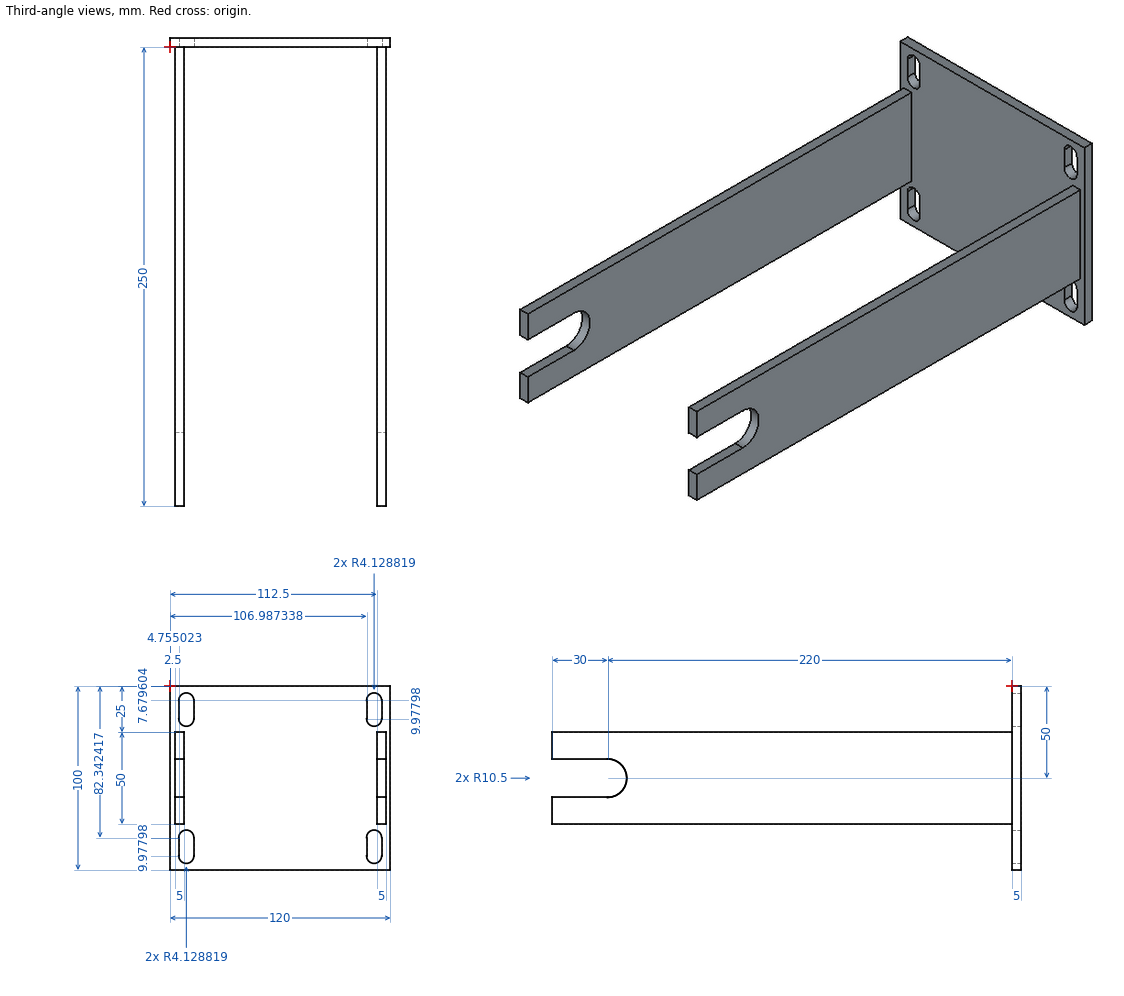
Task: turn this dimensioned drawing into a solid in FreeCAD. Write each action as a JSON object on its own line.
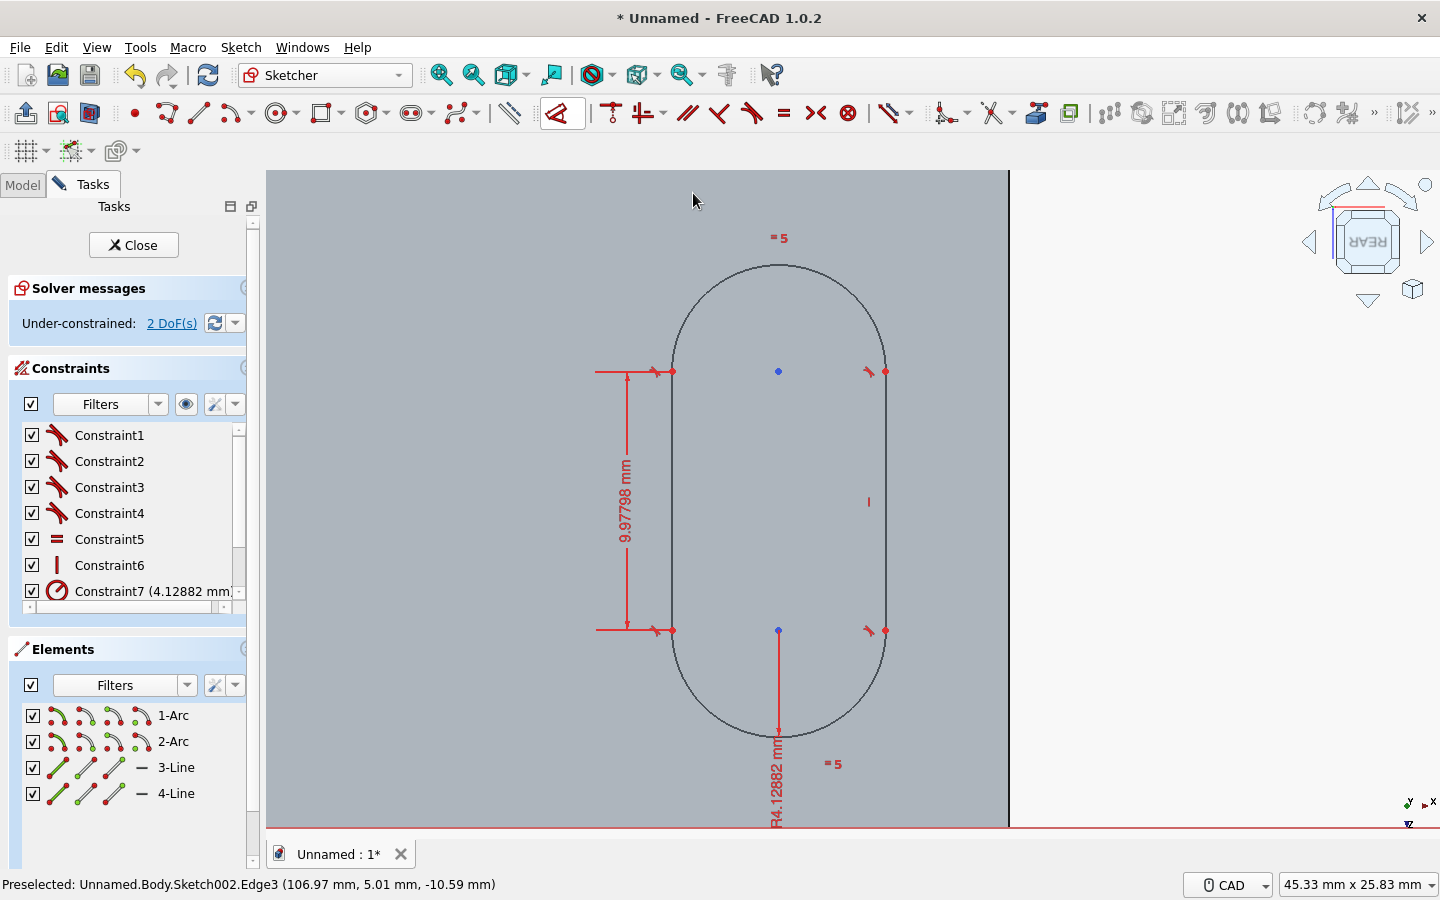
{"action": "left_click", "coordinate": [672, 630]}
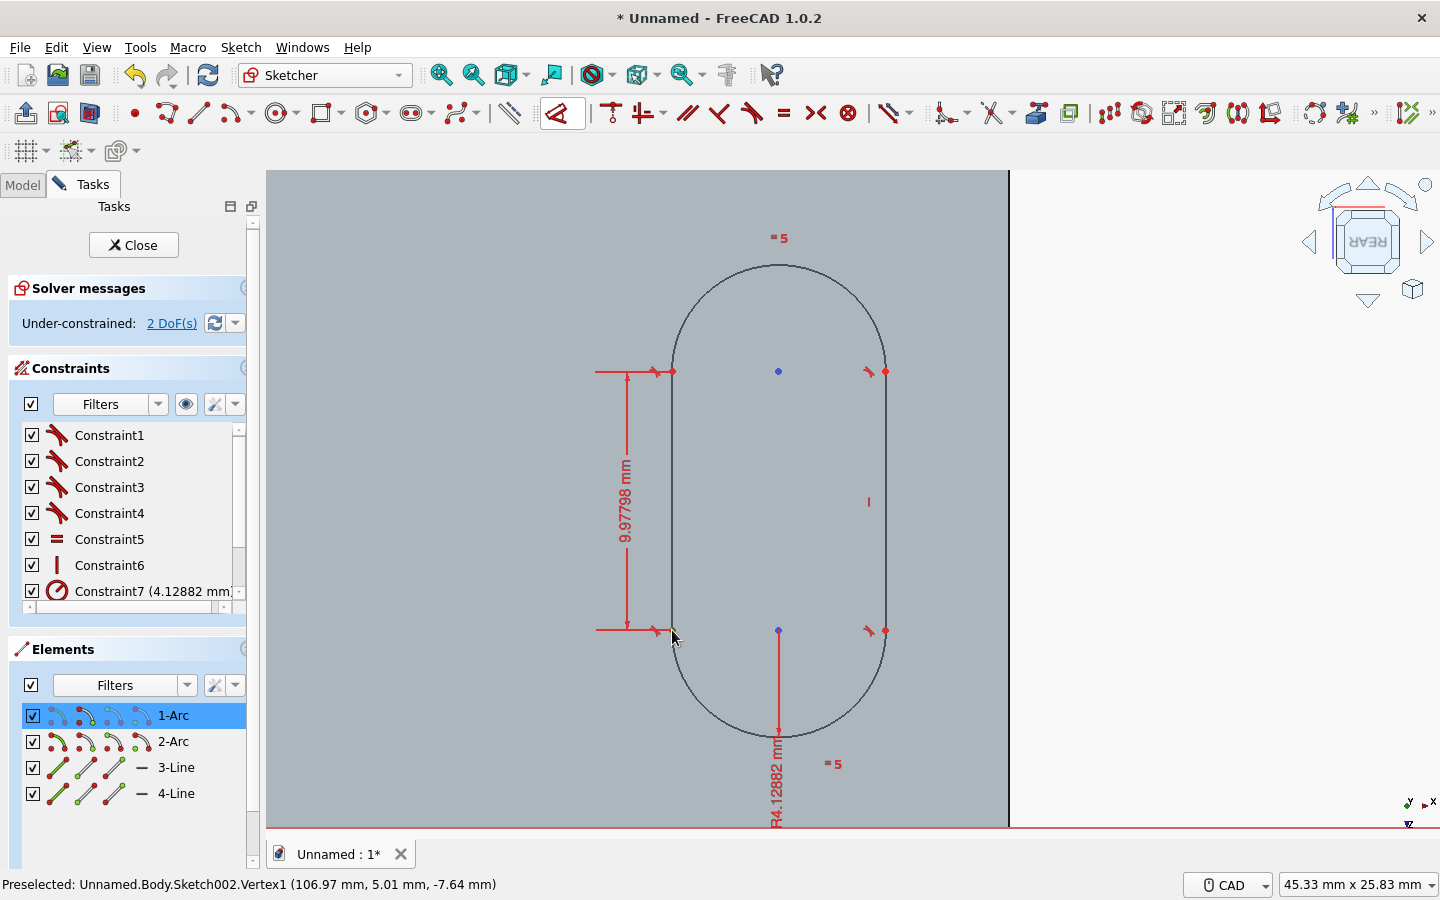
{"action": "left_click", "coordinate": [580, 114]}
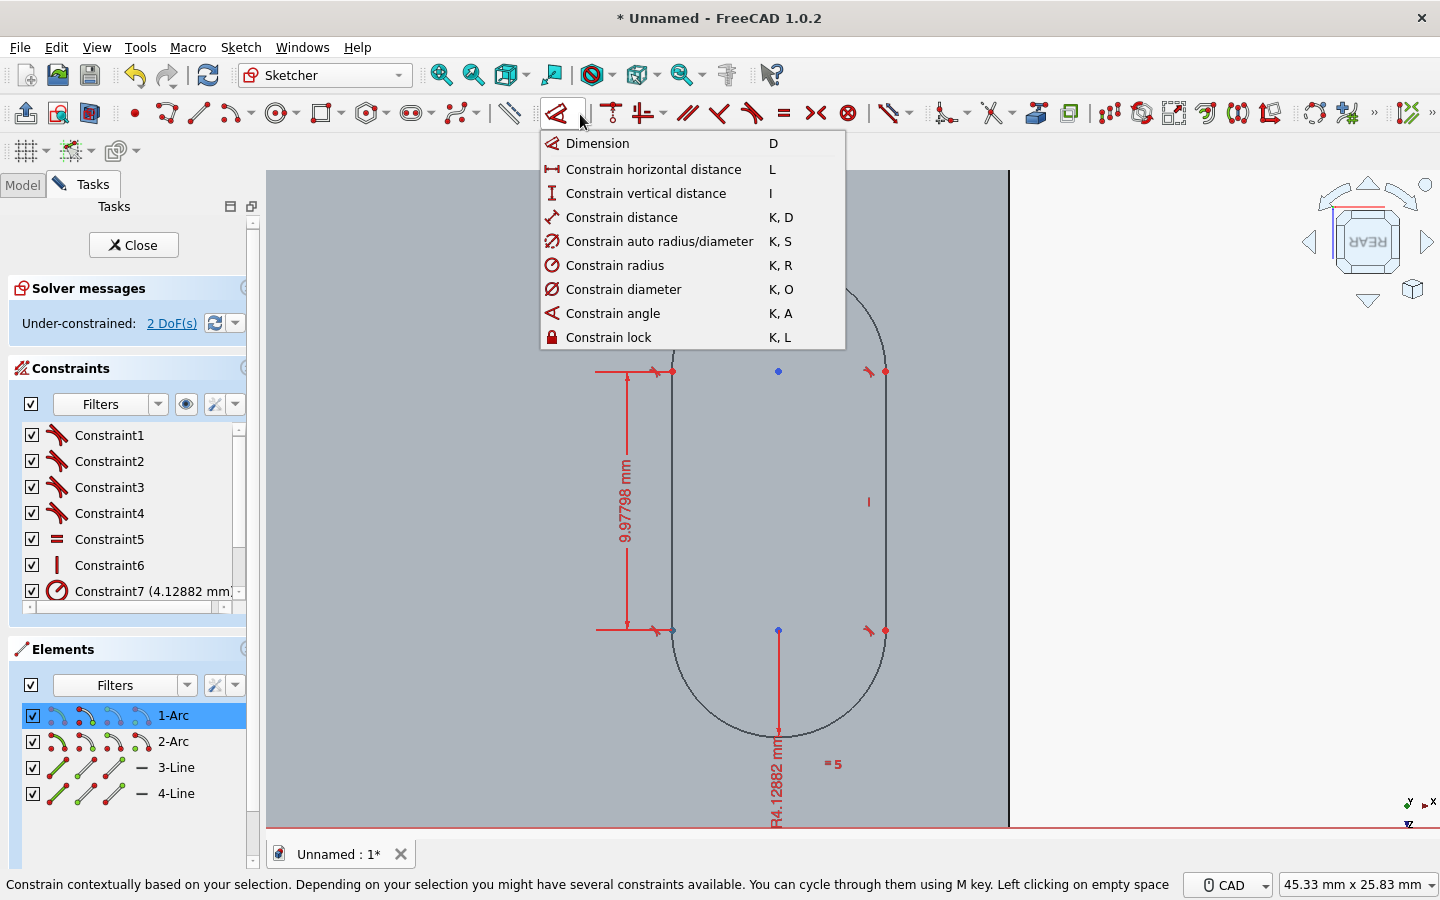
{"action": "left_click", "coordinate": [693, 193]}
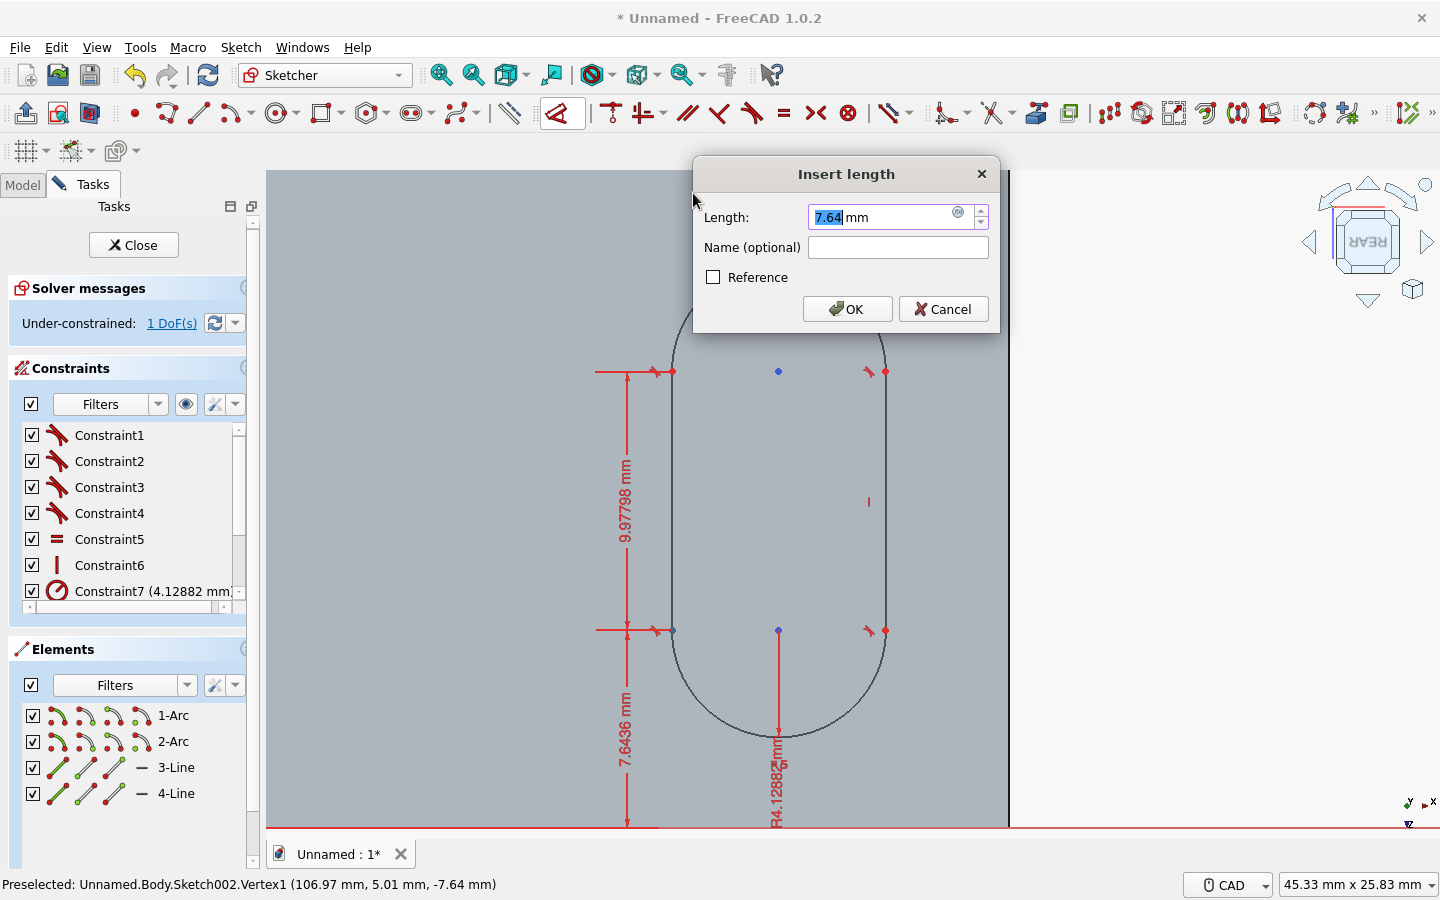
{"action": "type", "text": "7.679604"}
{"action": "key", "text": "Return"}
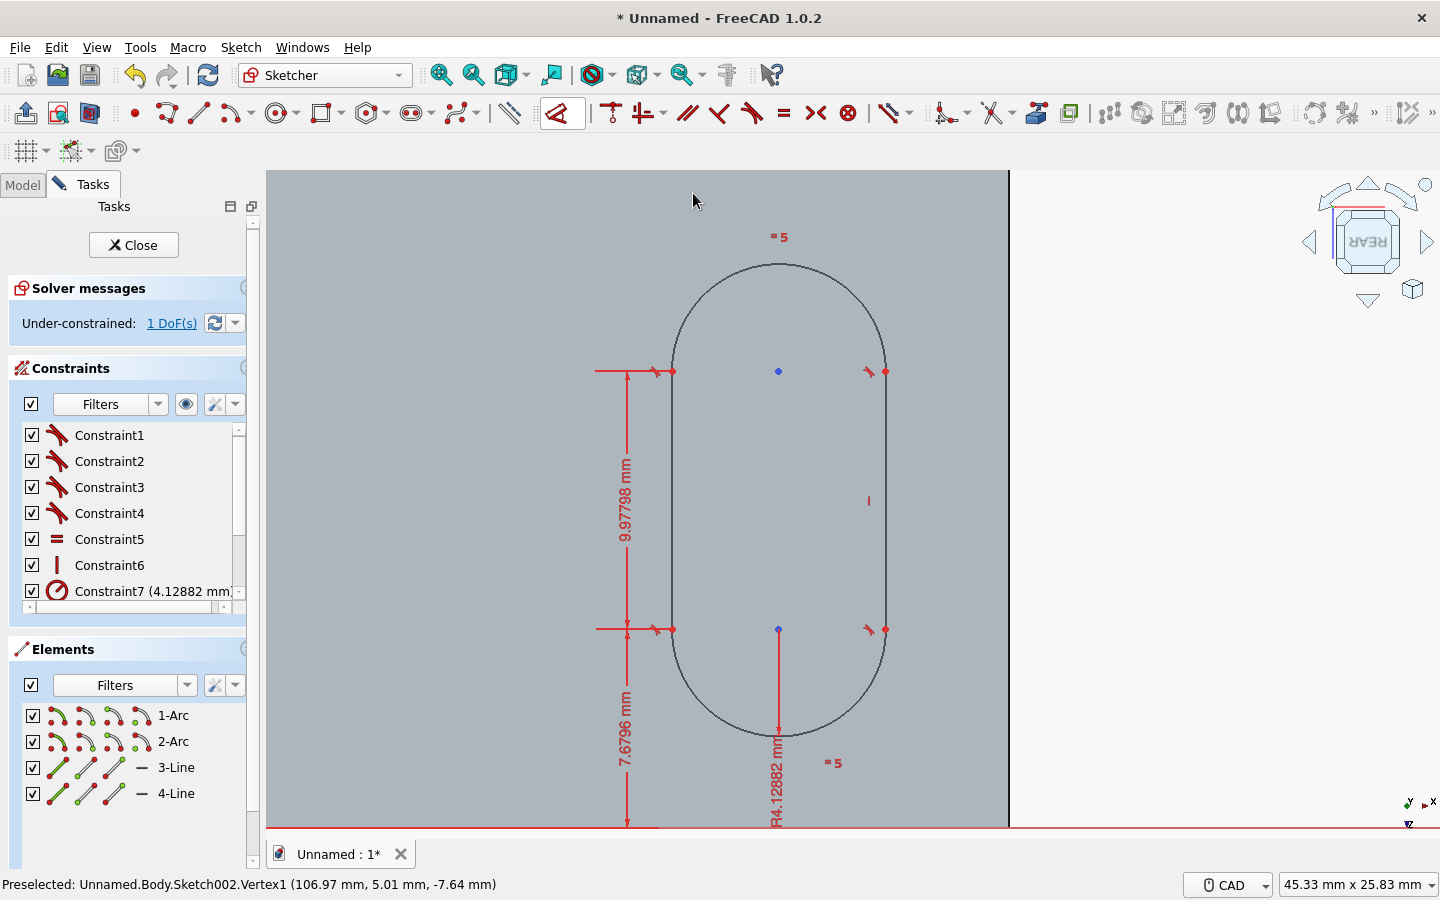
{"action": "left_click", "coordinate": [672, 629]}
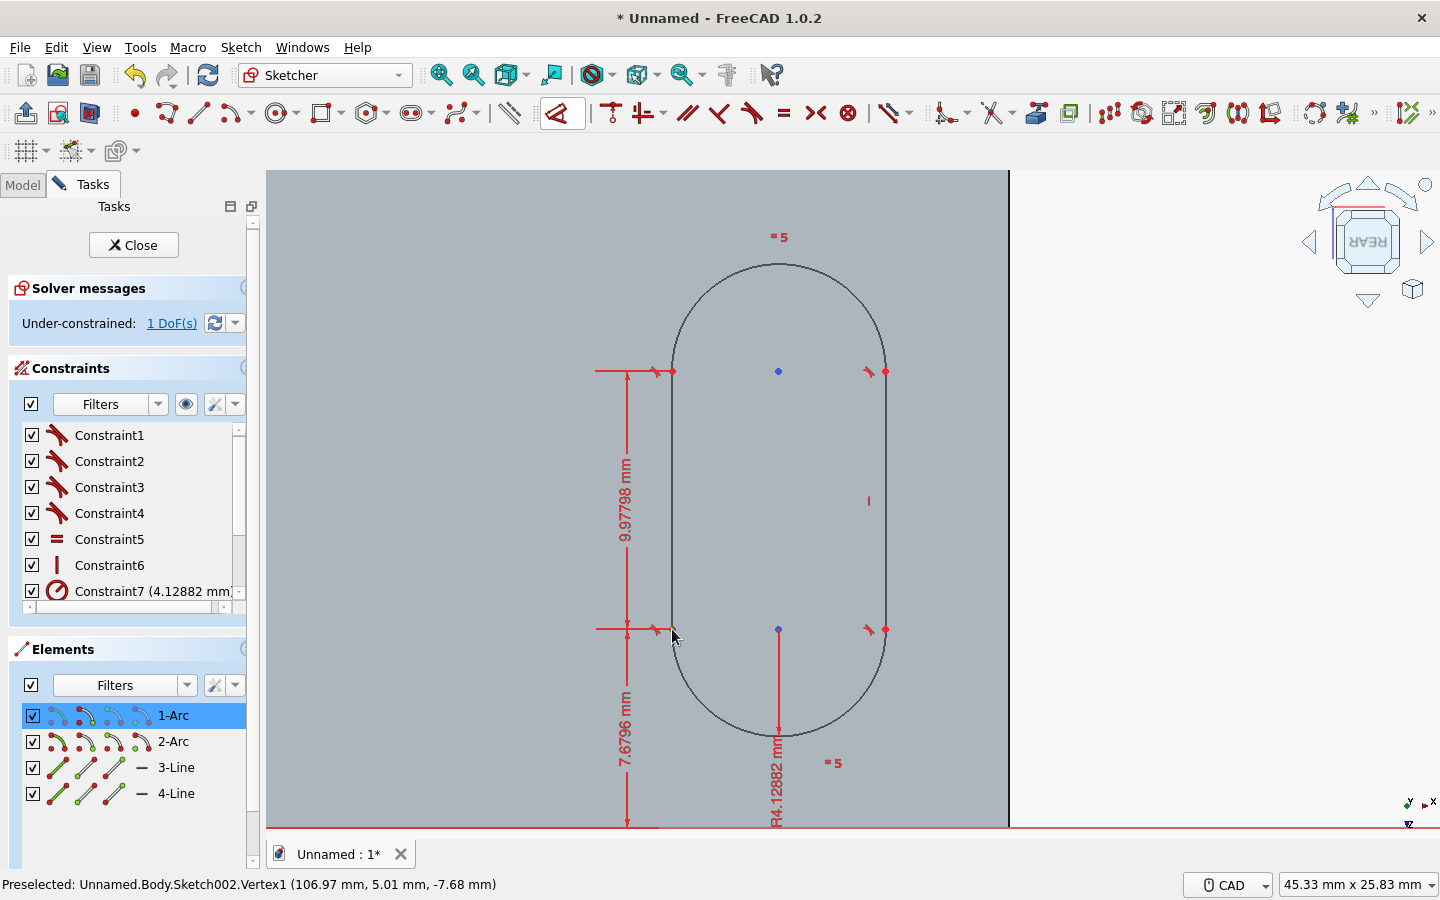
{"action": "key", "text": "l"}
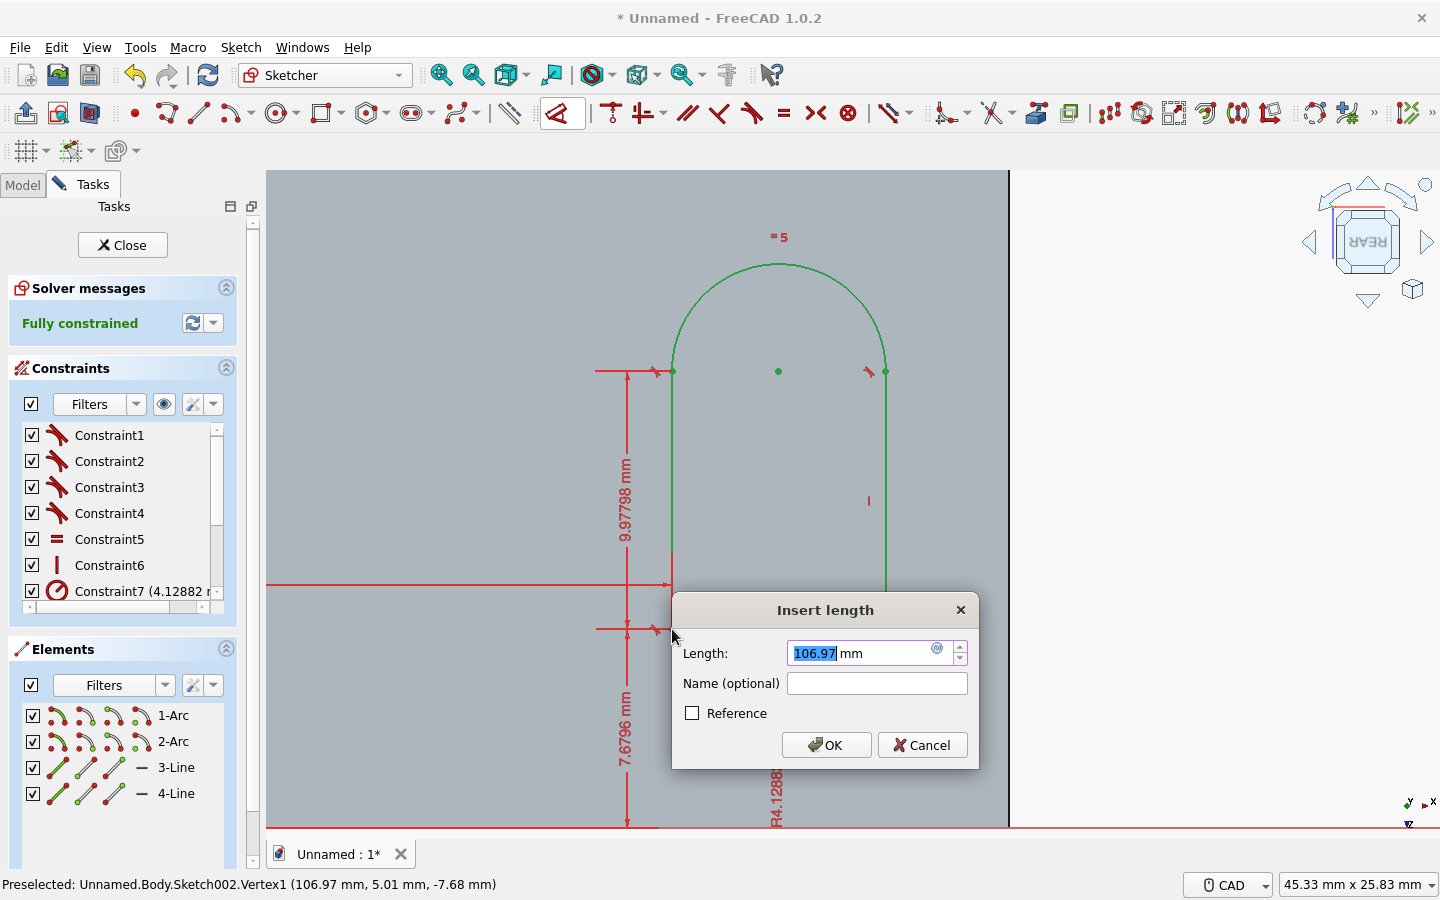
{"action": "type", "text": "106.987338"}
{"action": "key", "text": "Return"}